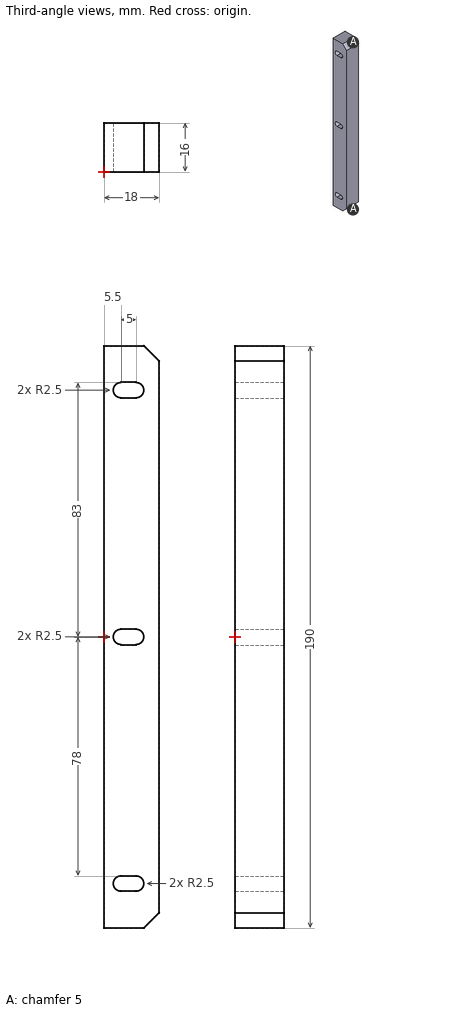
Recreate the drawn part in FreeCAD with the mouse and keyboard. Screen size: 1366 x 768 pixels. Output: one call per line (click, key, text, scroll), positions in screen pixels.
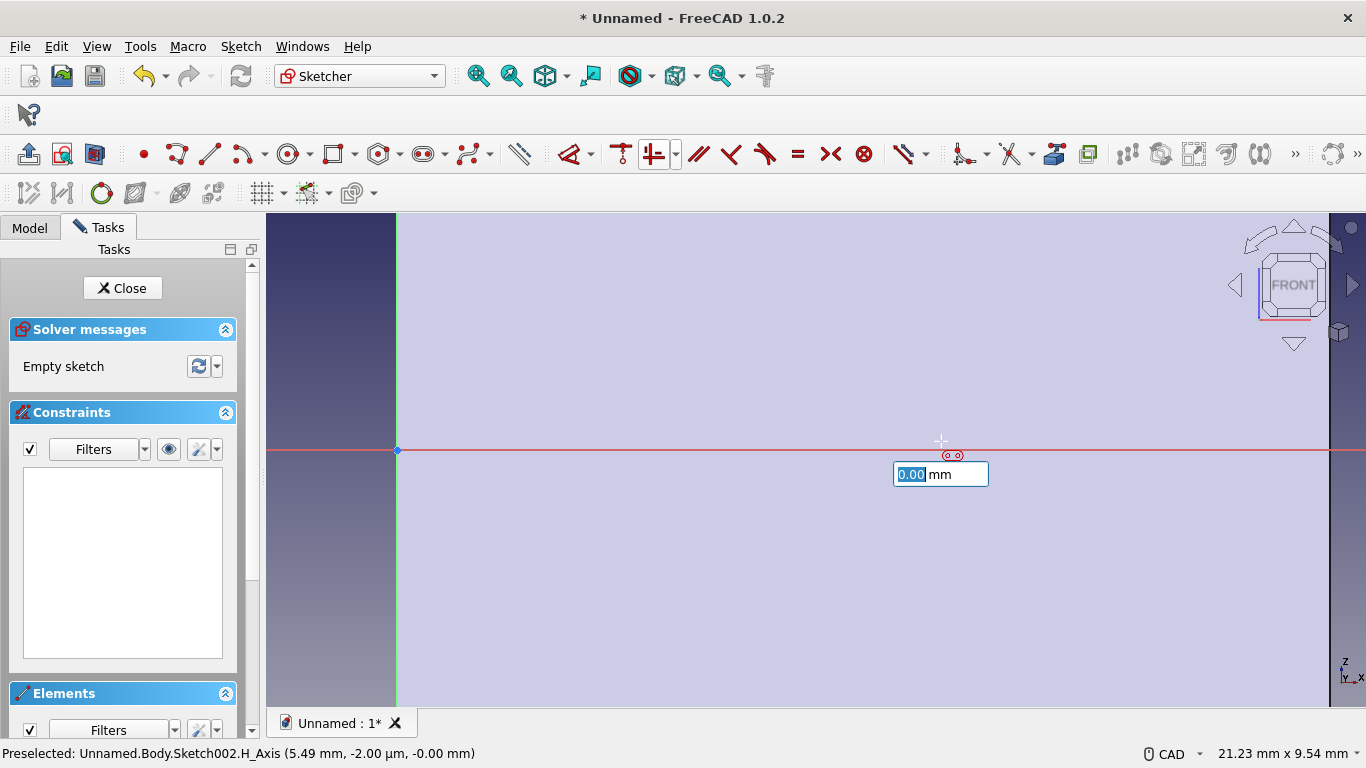
click(812, 321)
key(Escape)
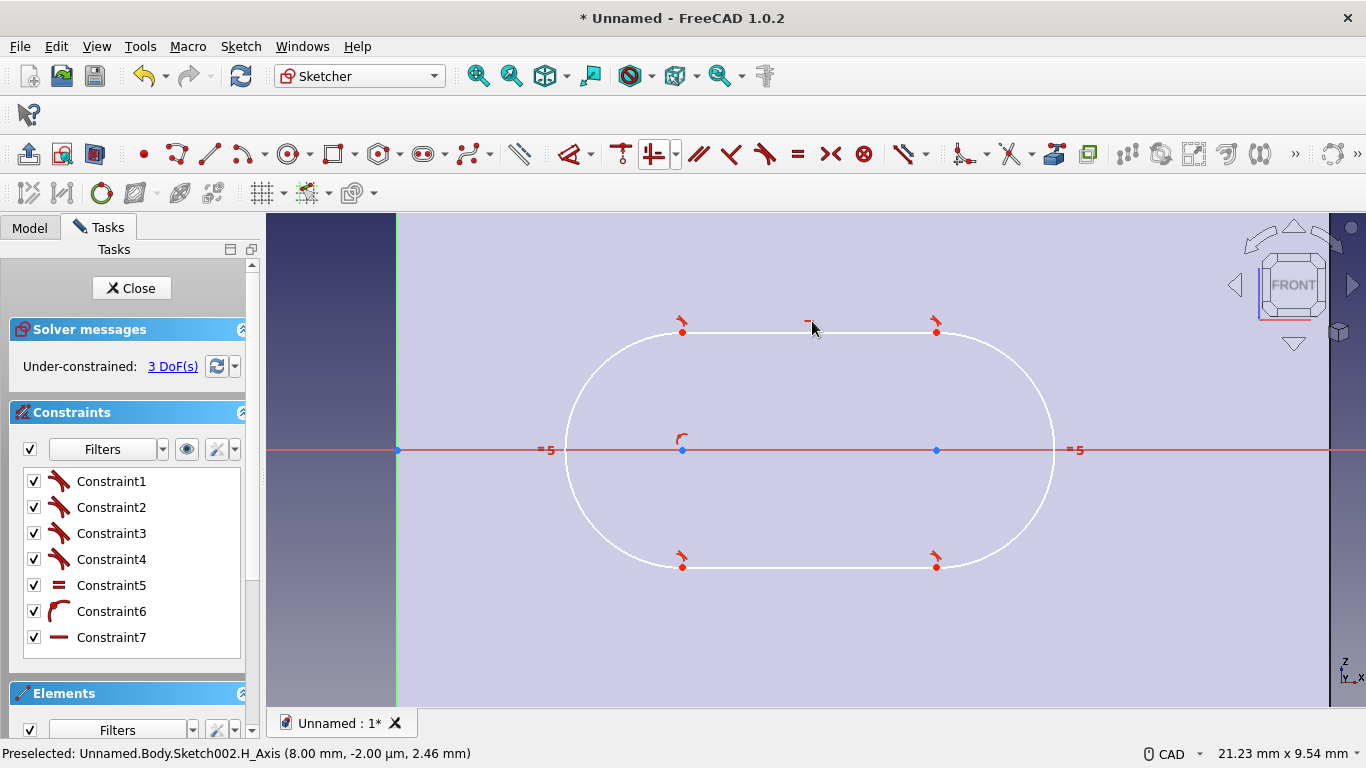
click(568, 154)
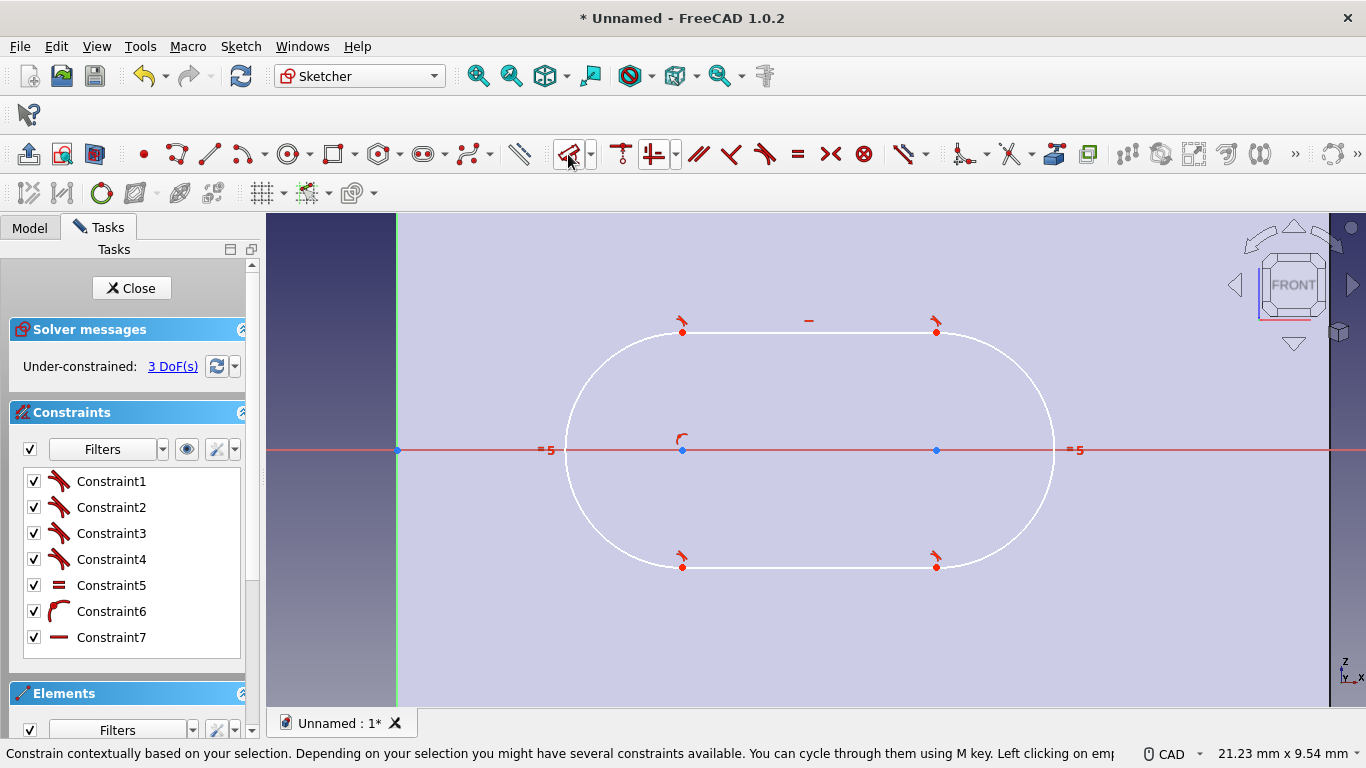
click(588, 381)
click(562, 362)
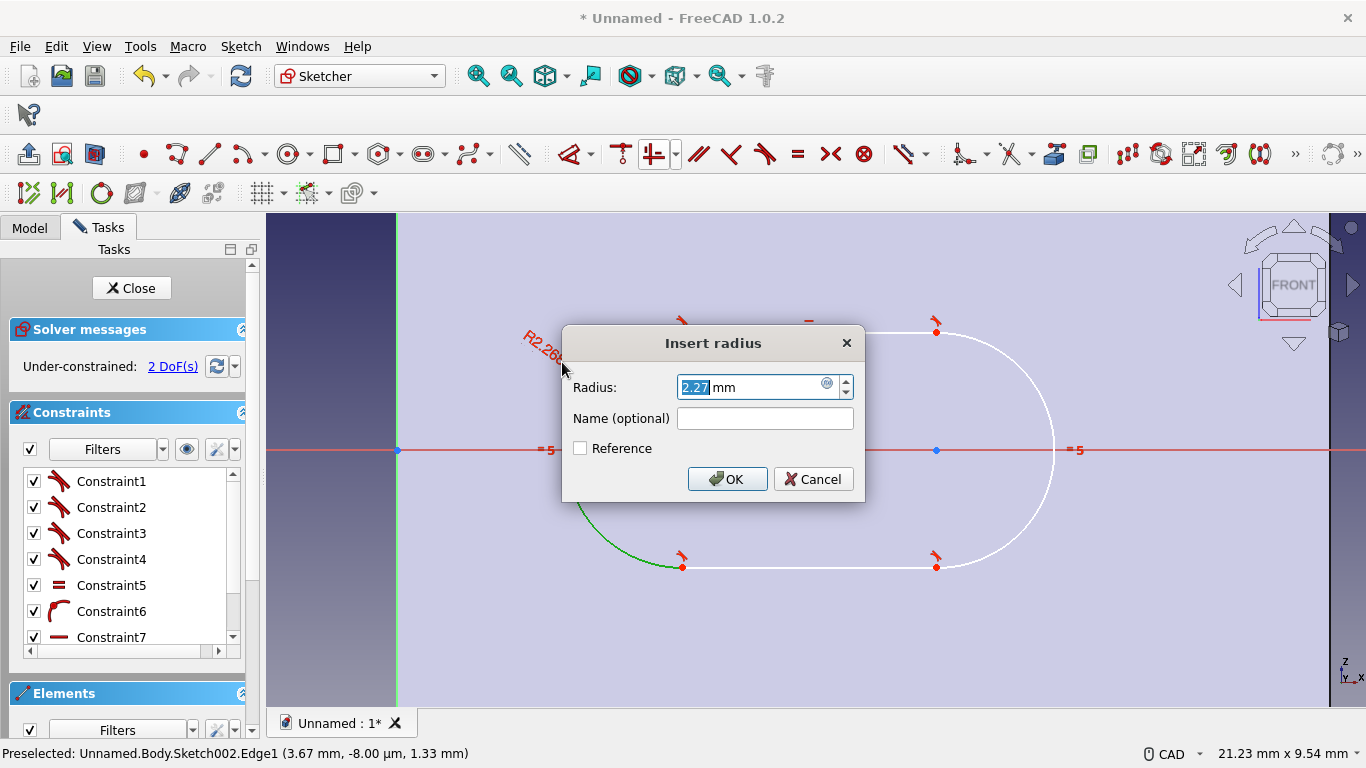
text(2.5)
key(Return)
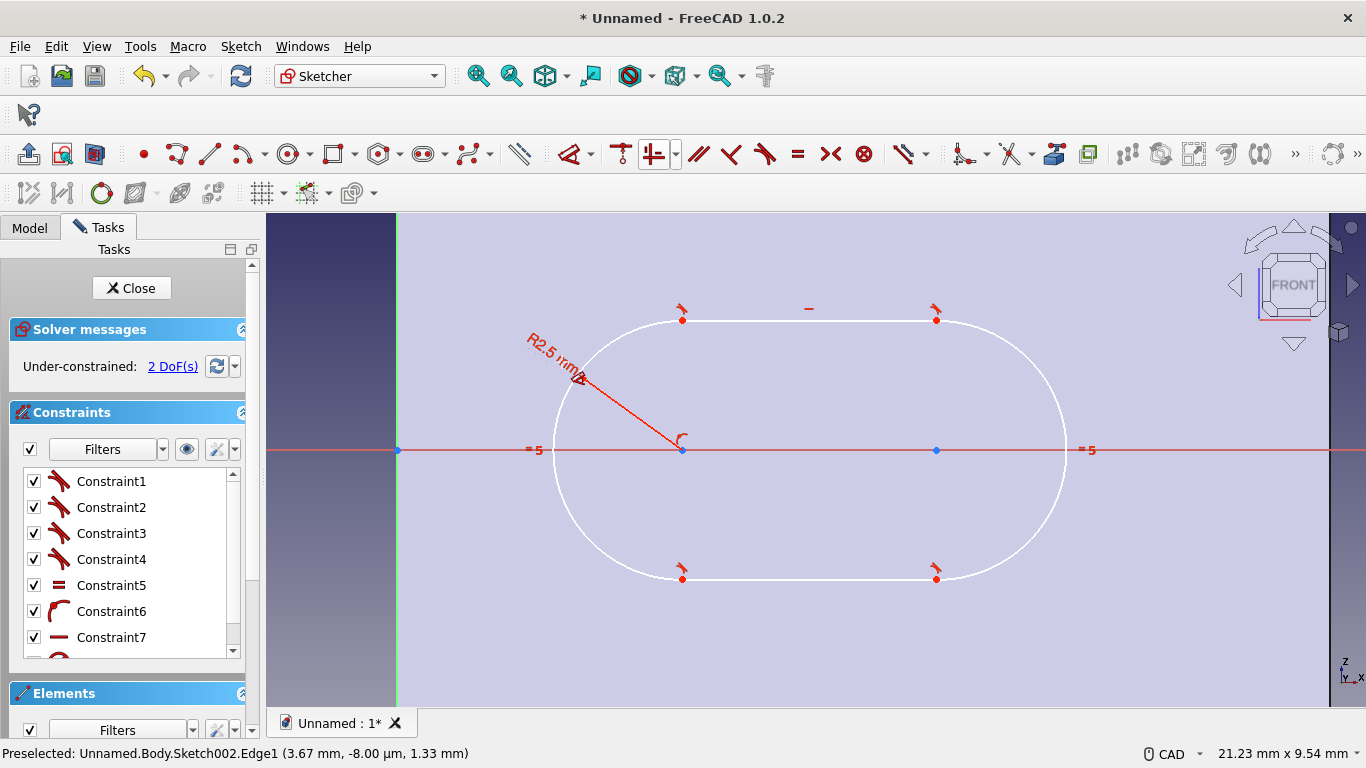
click(759, 321)
click(810, 287)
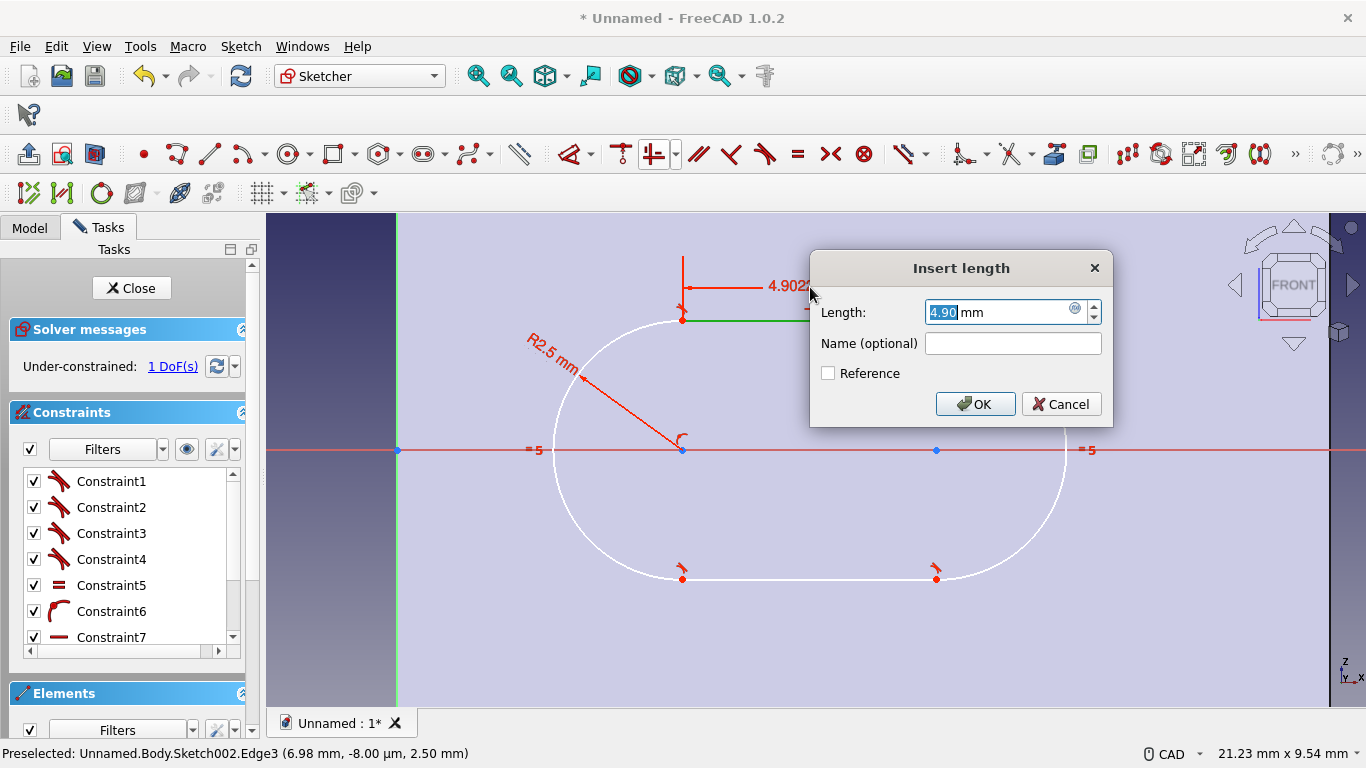
text(5)
key(Return)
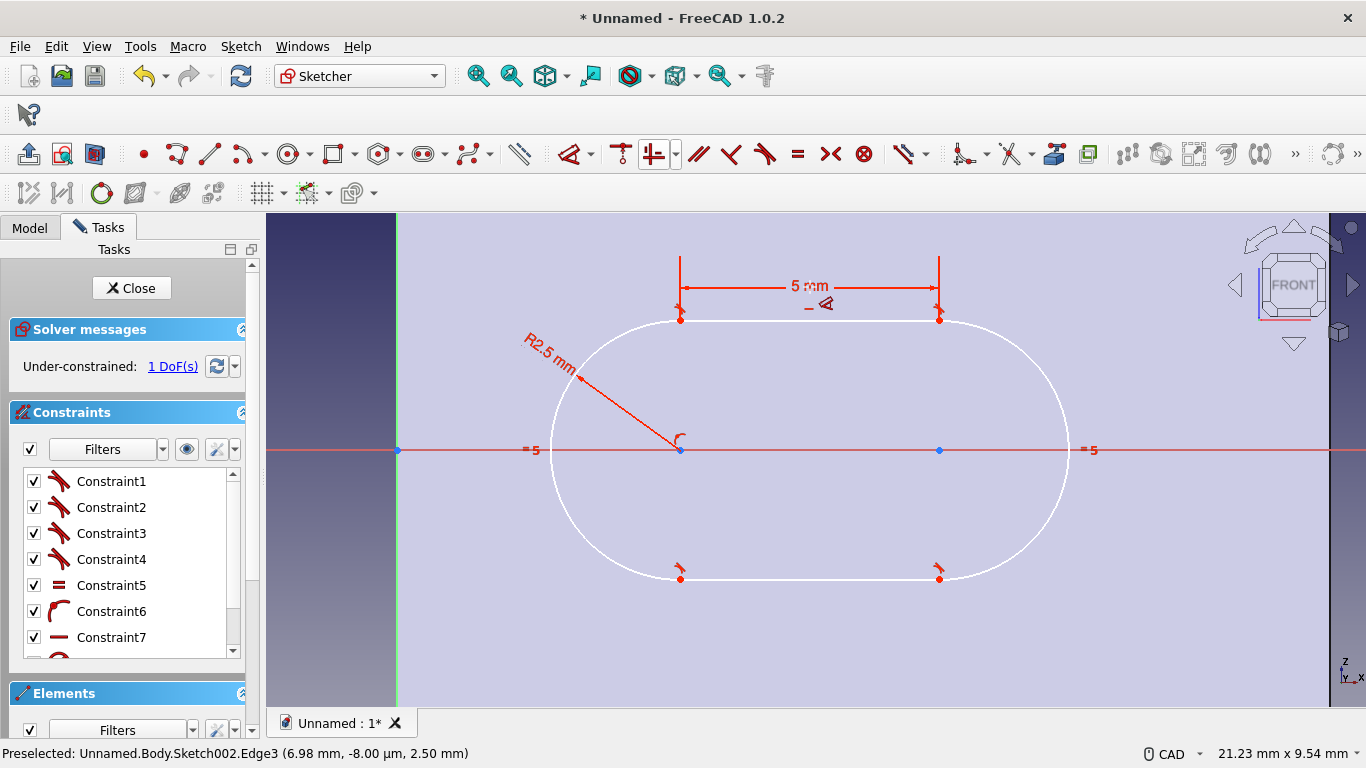
click(680, 321)
click(539, 287)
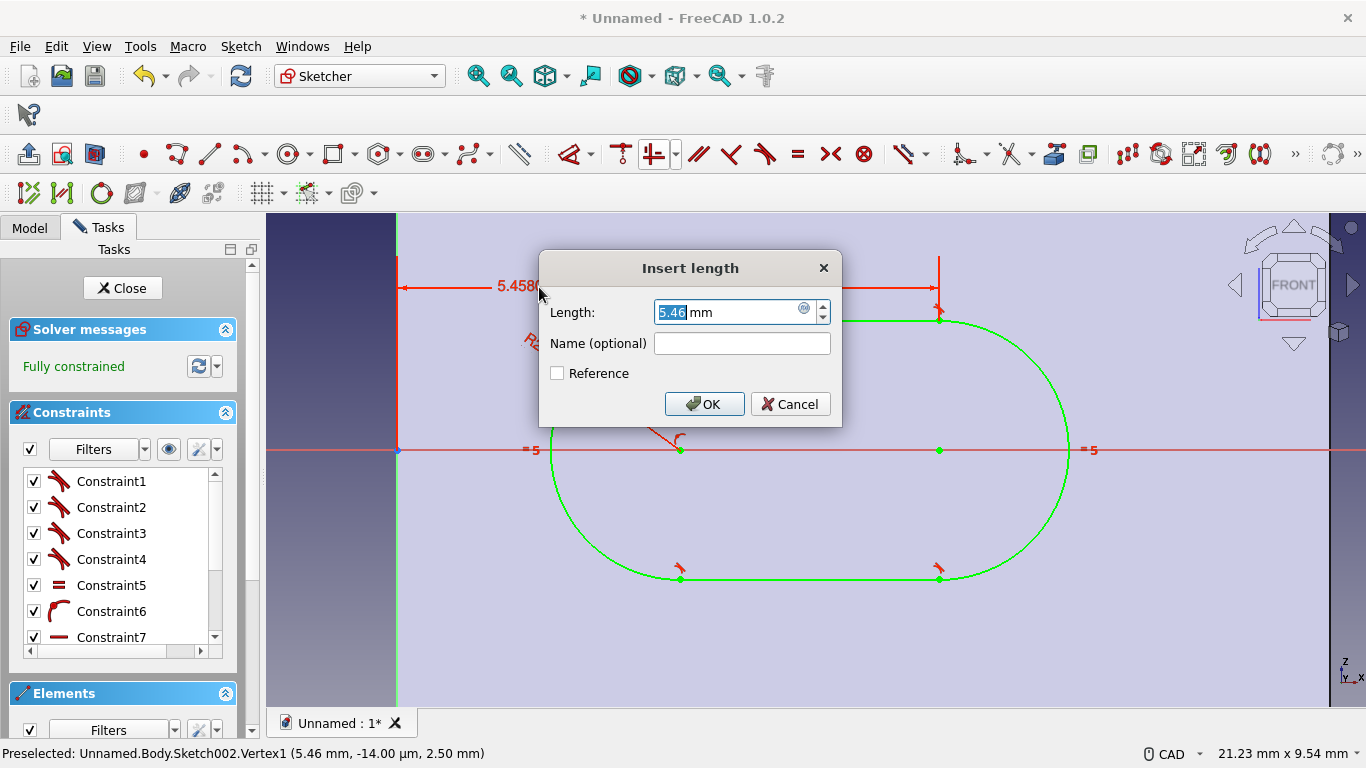
text(5.5)
key(Return)
key(Escape)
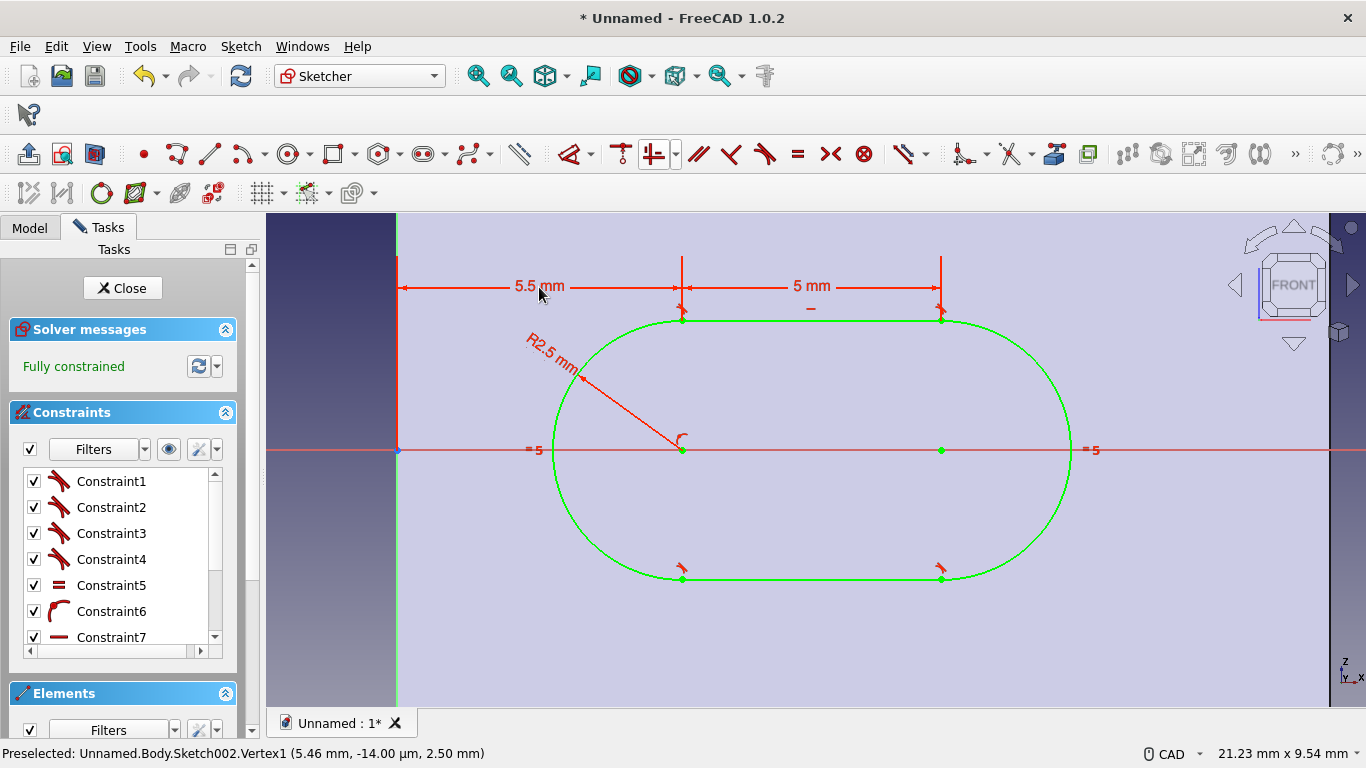
click(123, 288)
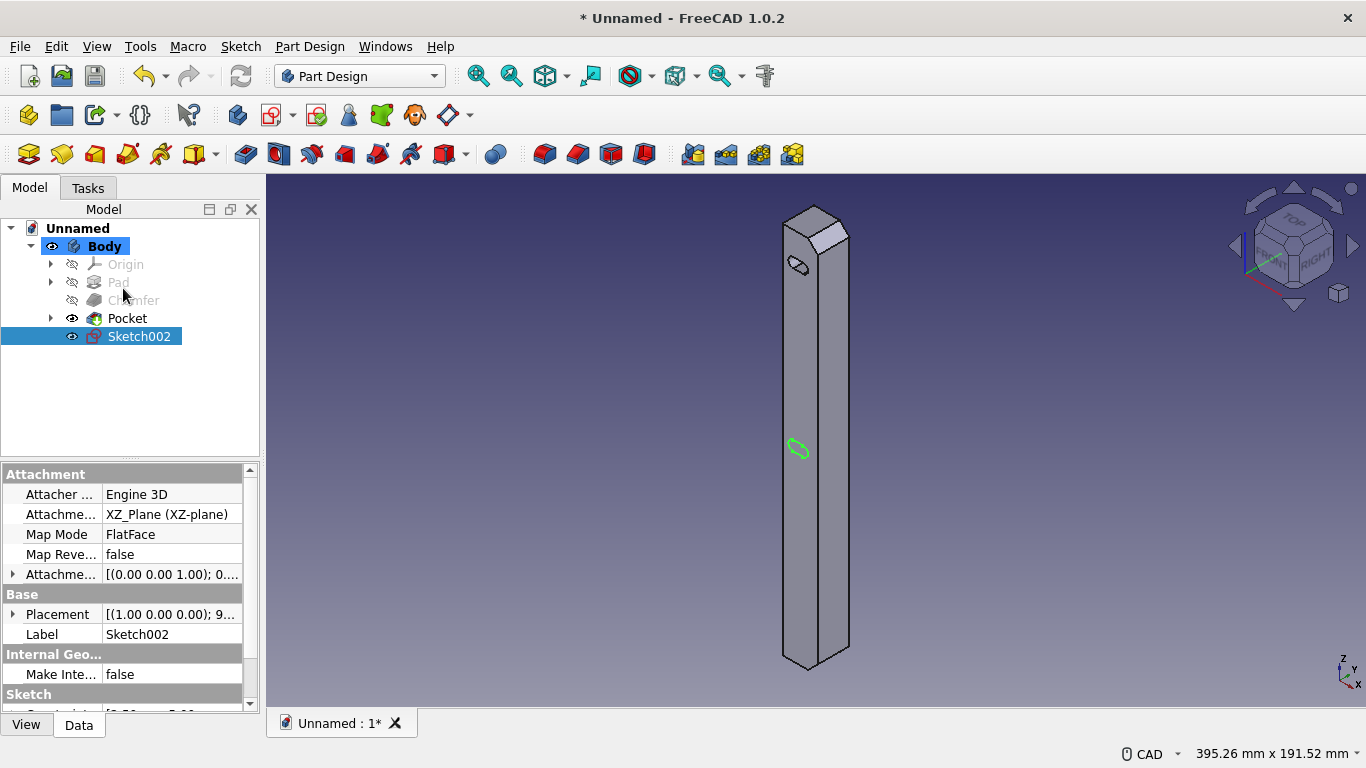
click(246, 154)